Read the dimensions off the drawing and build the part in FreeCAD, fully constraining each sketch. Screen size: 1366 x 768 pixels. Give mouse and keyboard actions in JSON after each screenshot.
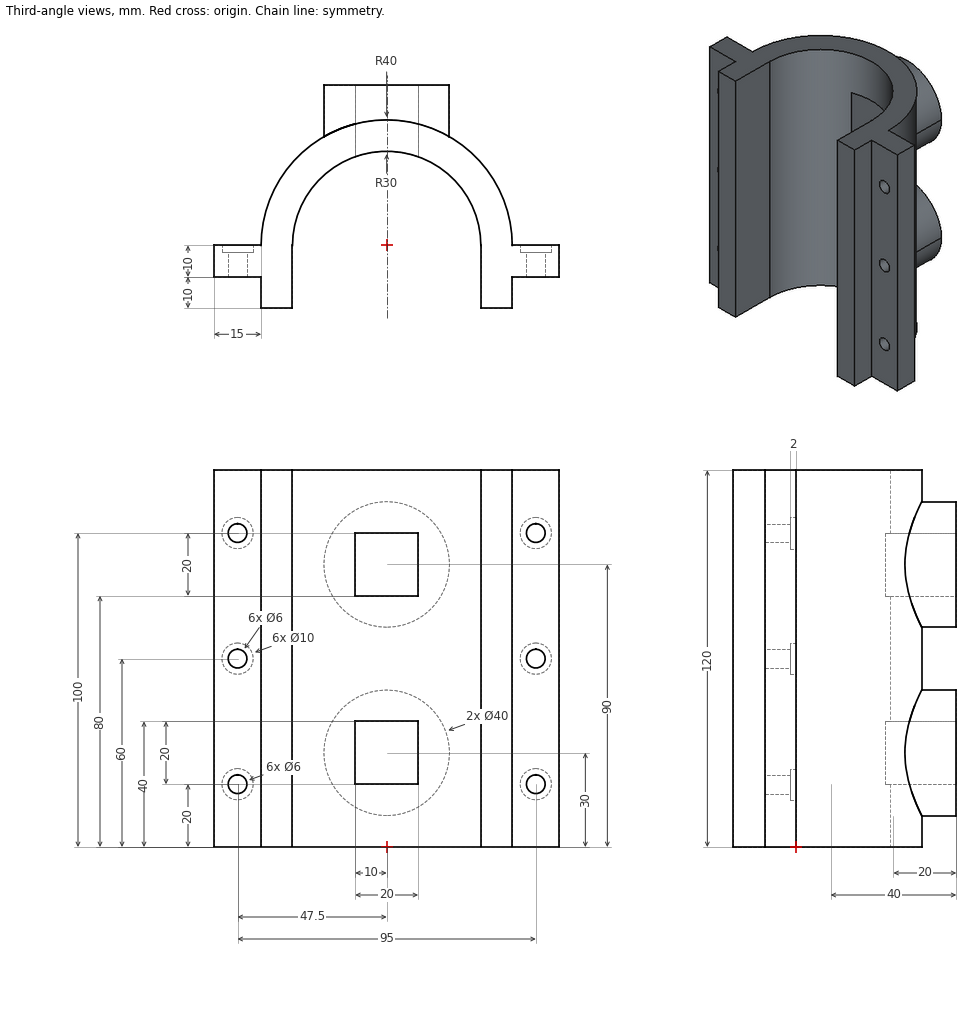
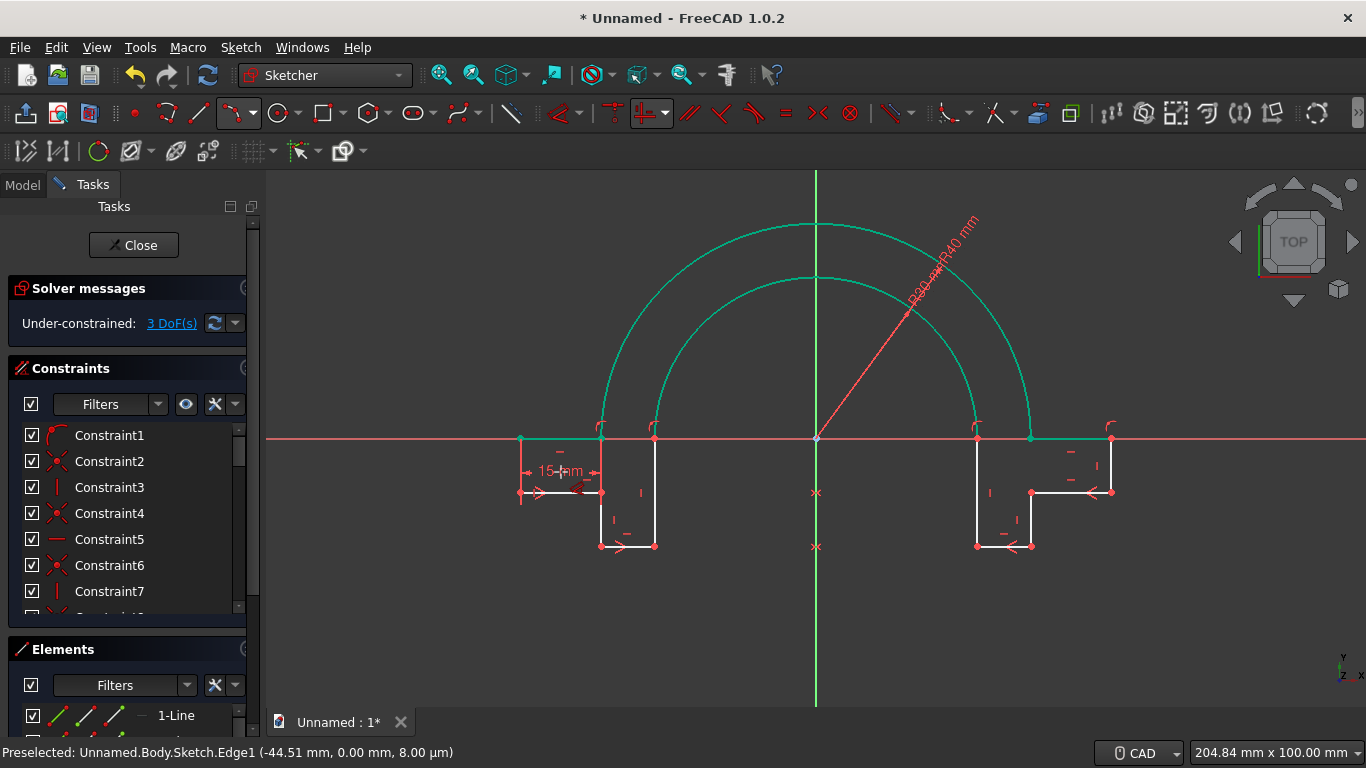
{"action": "left_click", "coordinate": [521, 455]}
{"action": "left_click", "coordinate": [487, 466]}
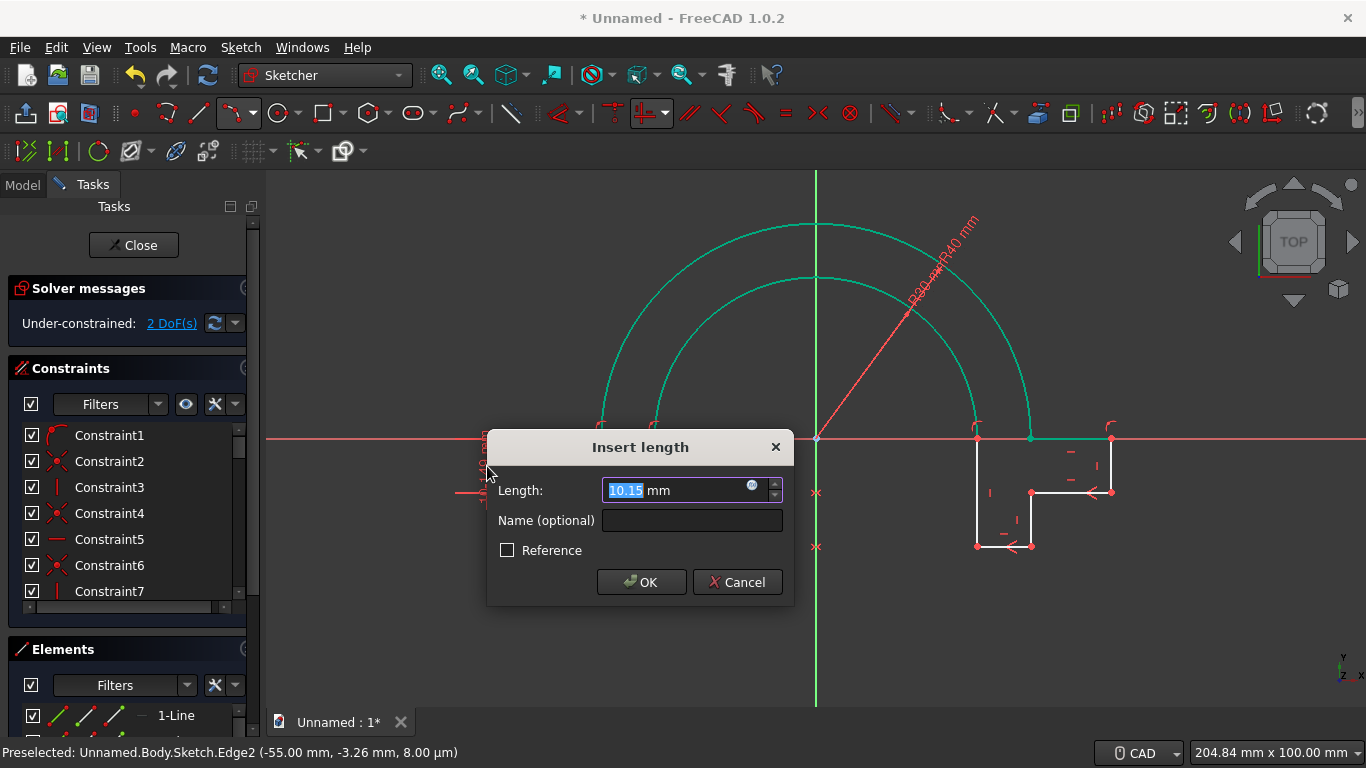
{"action": "type", "text": "10"}
{"action": "key", "text": "Return"}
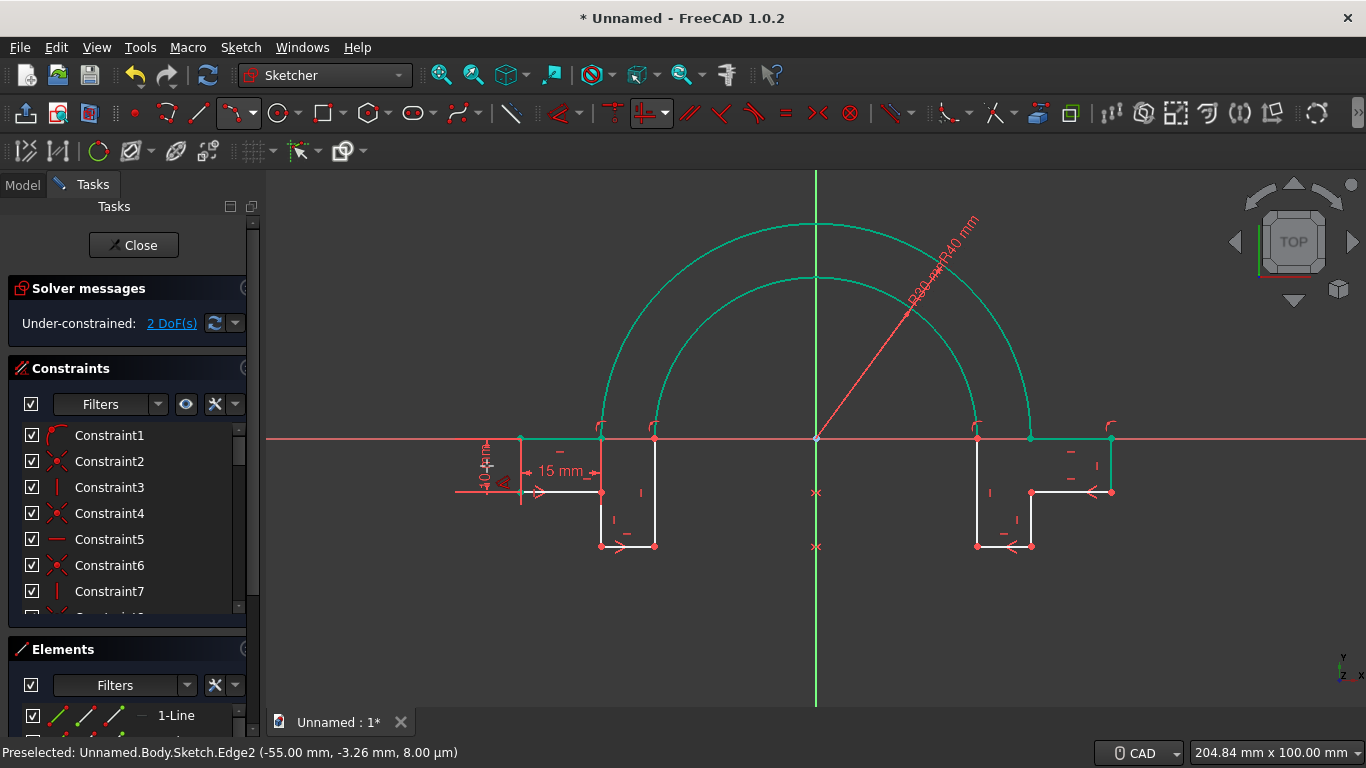
{"action": "left_click", "coordinate": [545, 492]}
{"action": "left_click", "coordinate": [561, 526]}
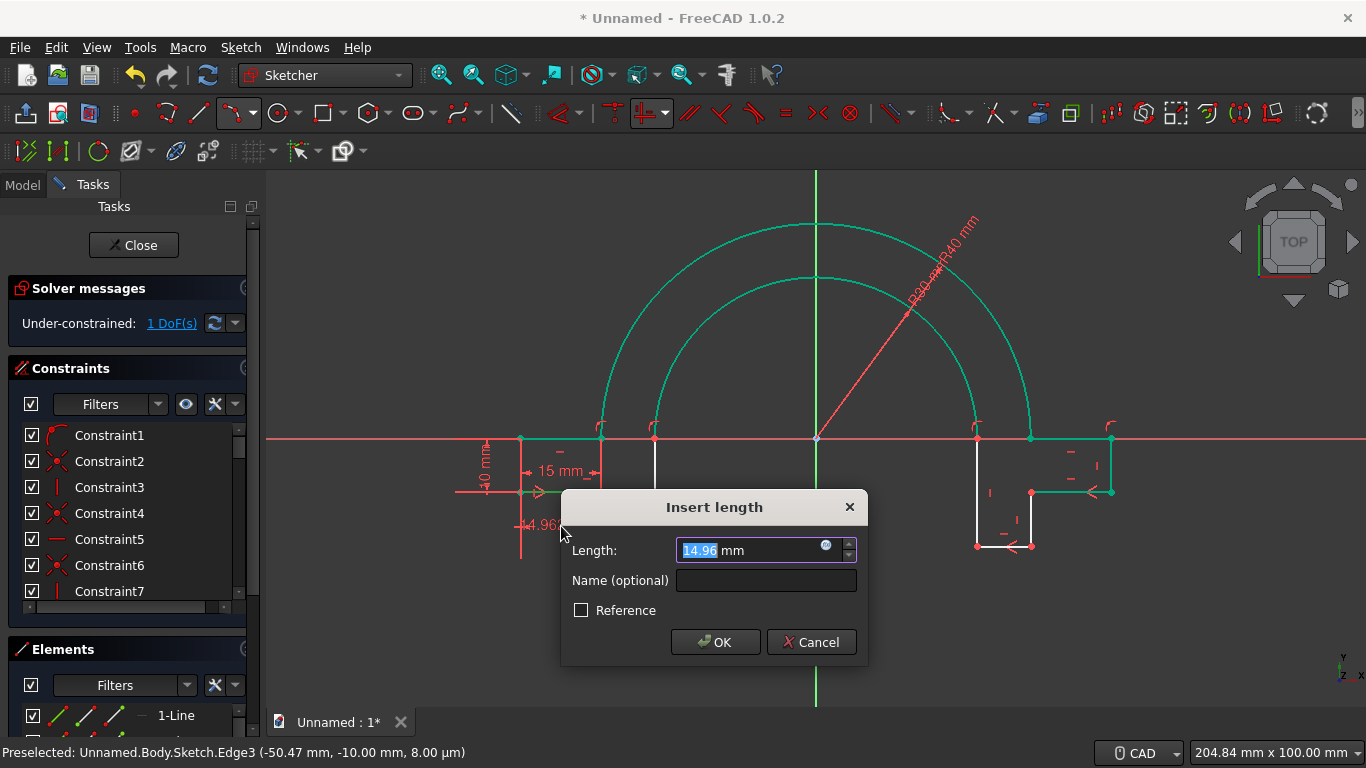
{"action": "type", "text": "15"}
{"action": "key", "text": "Return"}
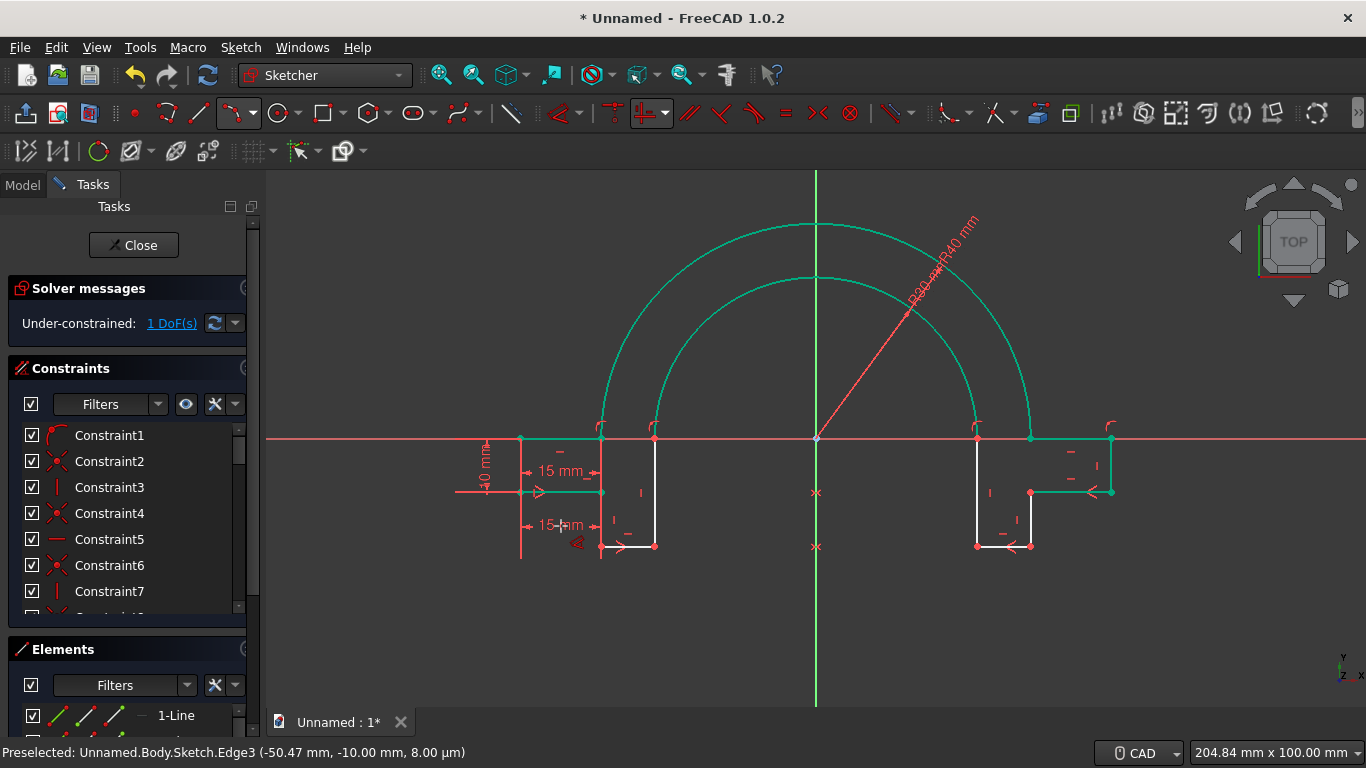
{"action": "left_click", "coordinate": [601, 509]}
{"action": "left_click", "coordinate": [635, 520]}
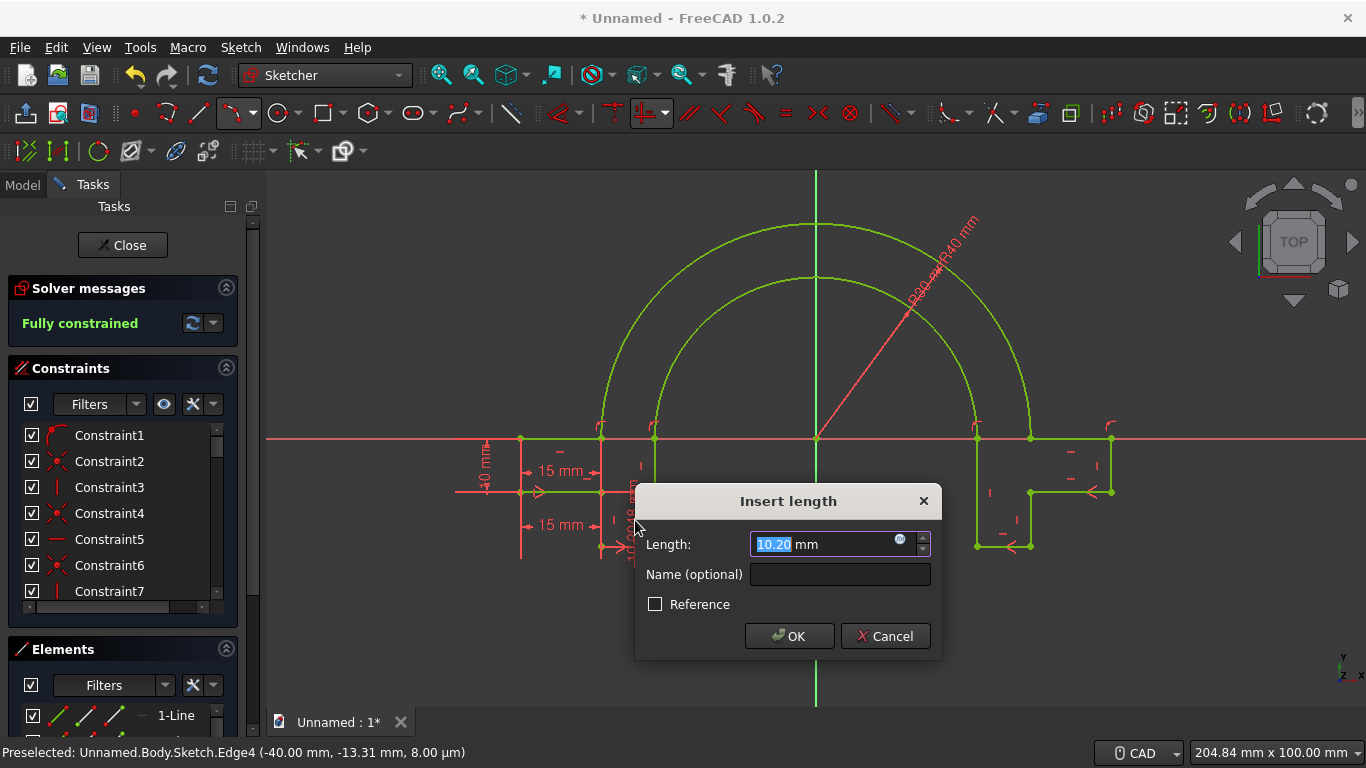
{"action": "type", "text": "10"}
{"action": "key", "text": "Return"}
{"action": "key", "text": "Escape"}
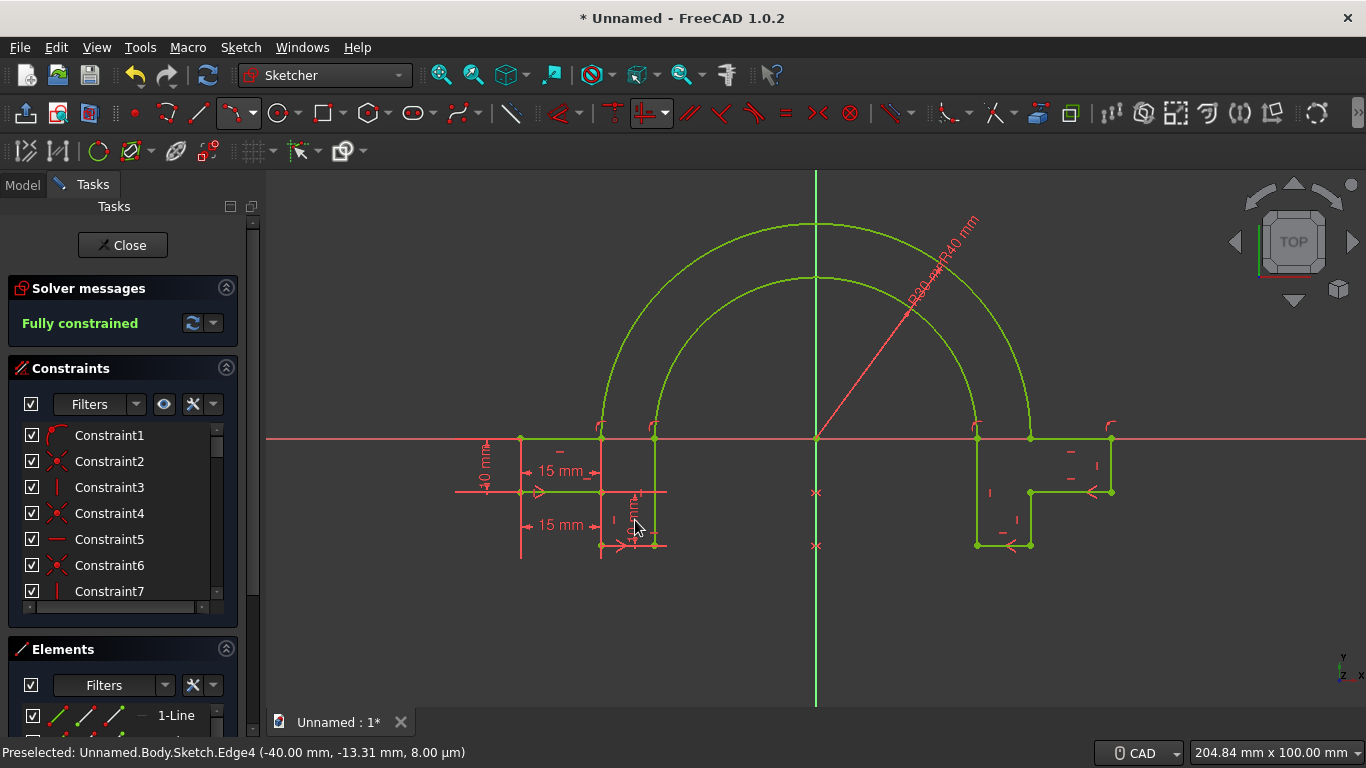
{"action": "left_click", "coordinate": [123, 245]}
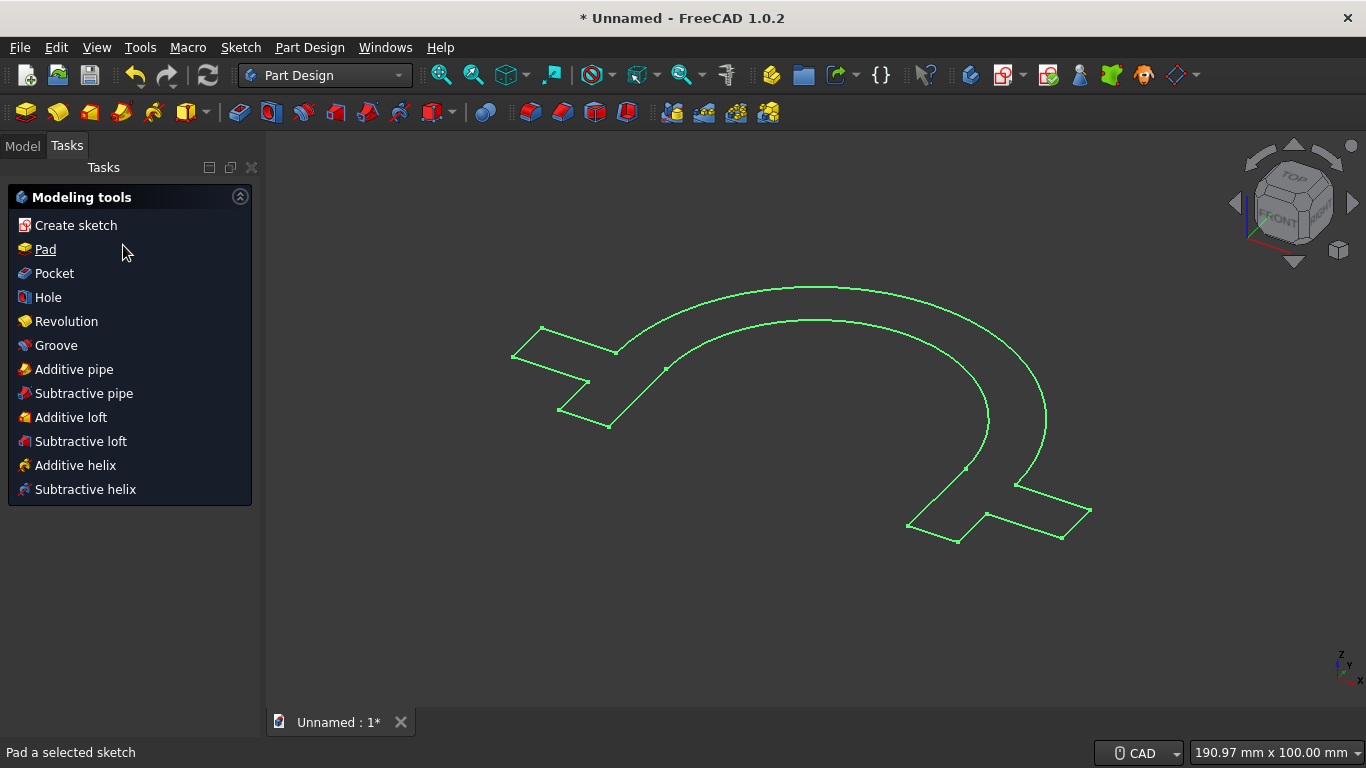
{"action": "left_click", "coordinate": [26, 112]}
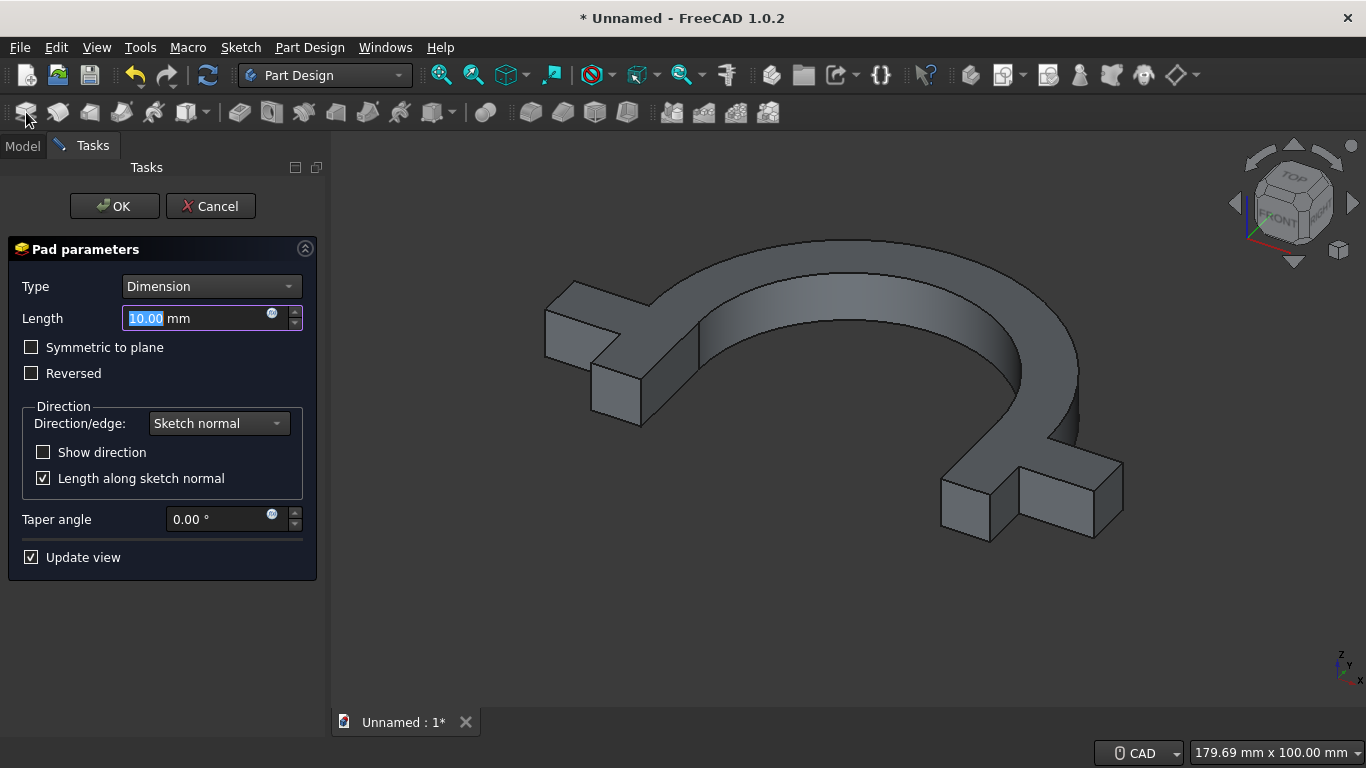
{"action": "type", "text": "120"}
{"action": "key", "text": "Tab"}